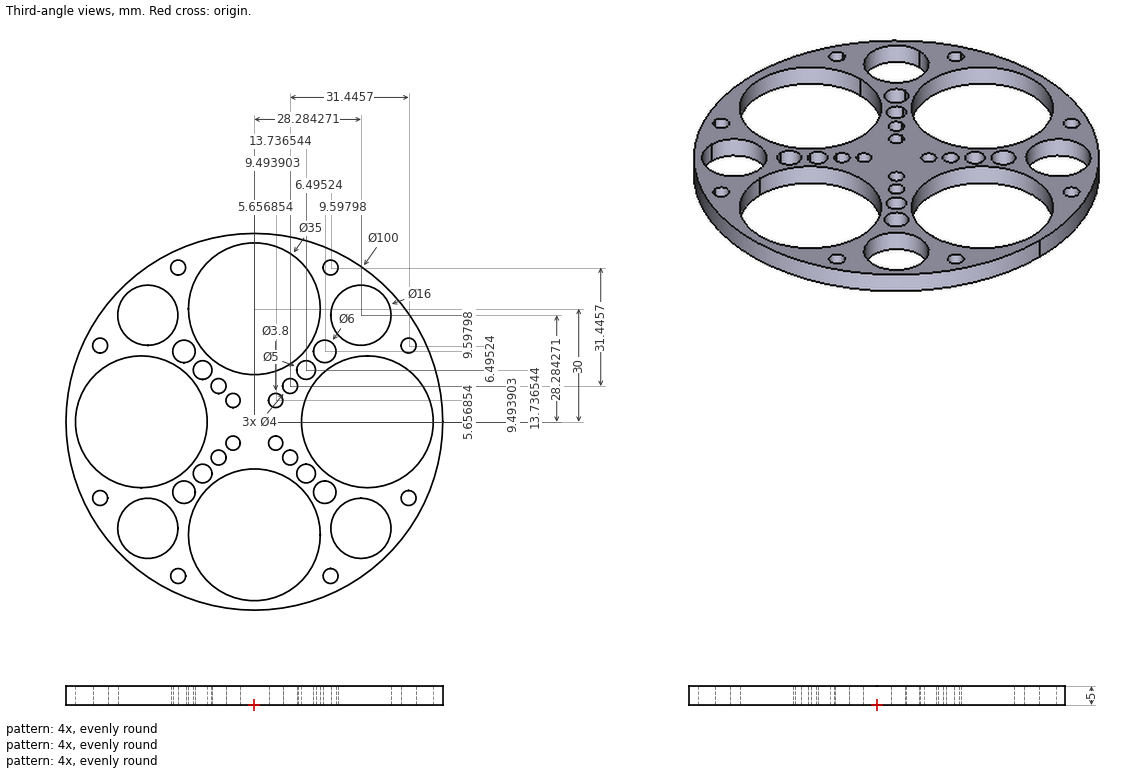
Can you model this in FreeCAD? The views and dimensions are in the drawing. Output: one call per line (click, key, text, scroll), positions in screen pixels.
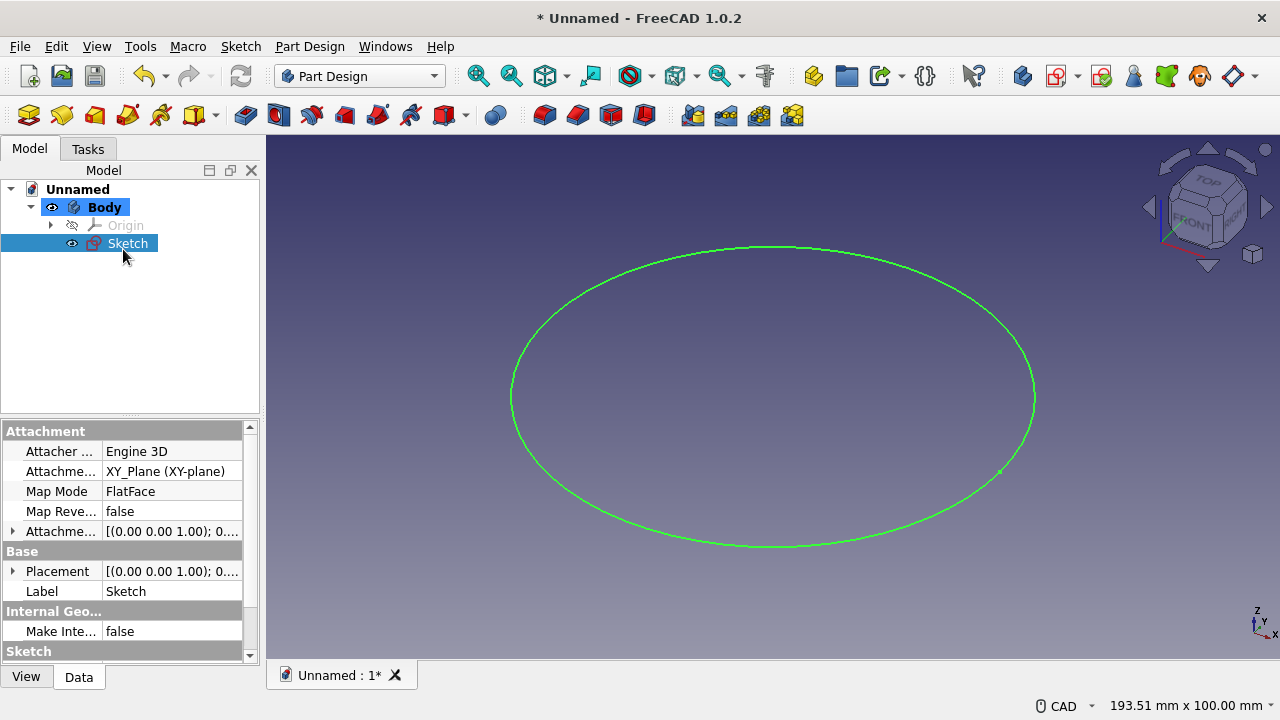
click(29, 116)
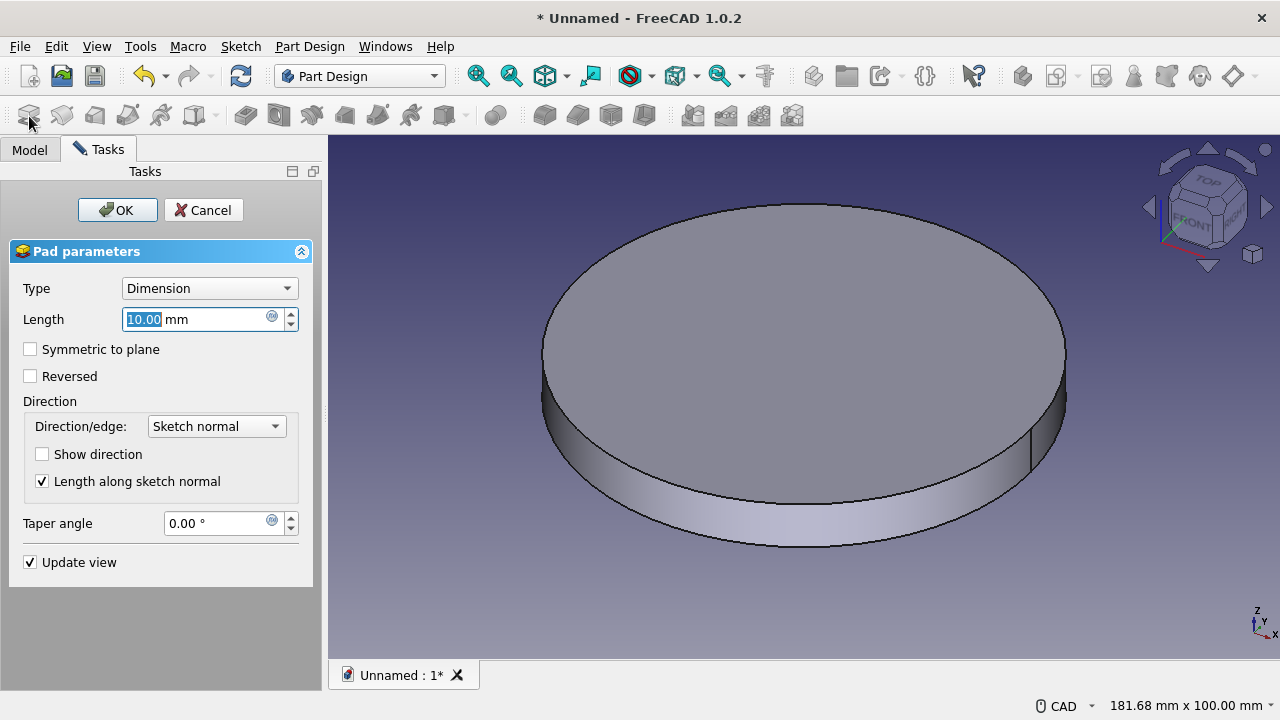
text(5)
key(Tab)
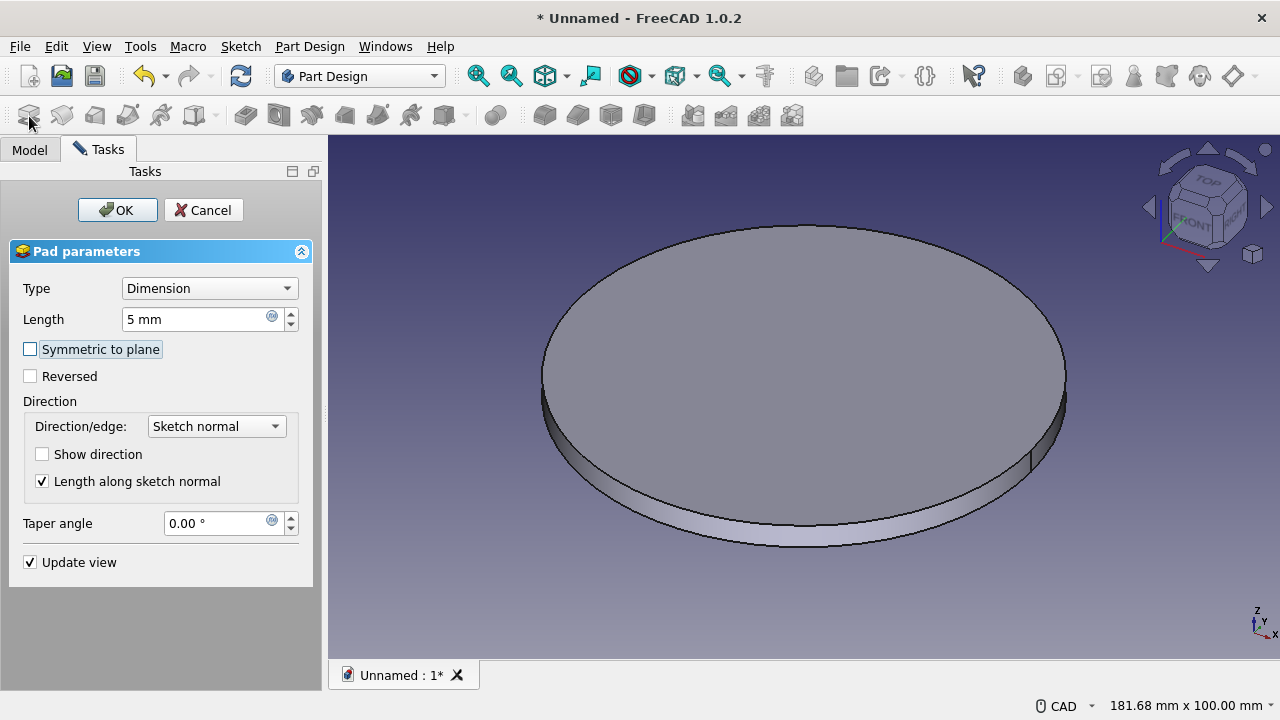
click(118, 210)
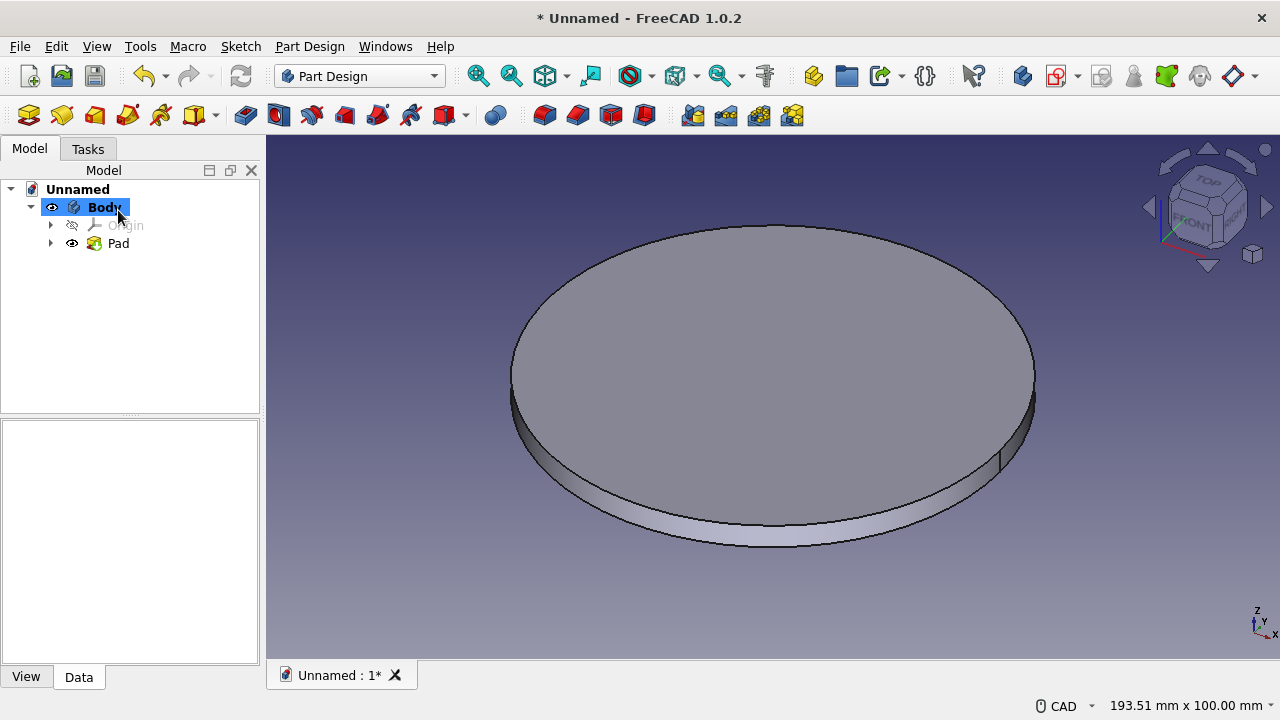
key(5)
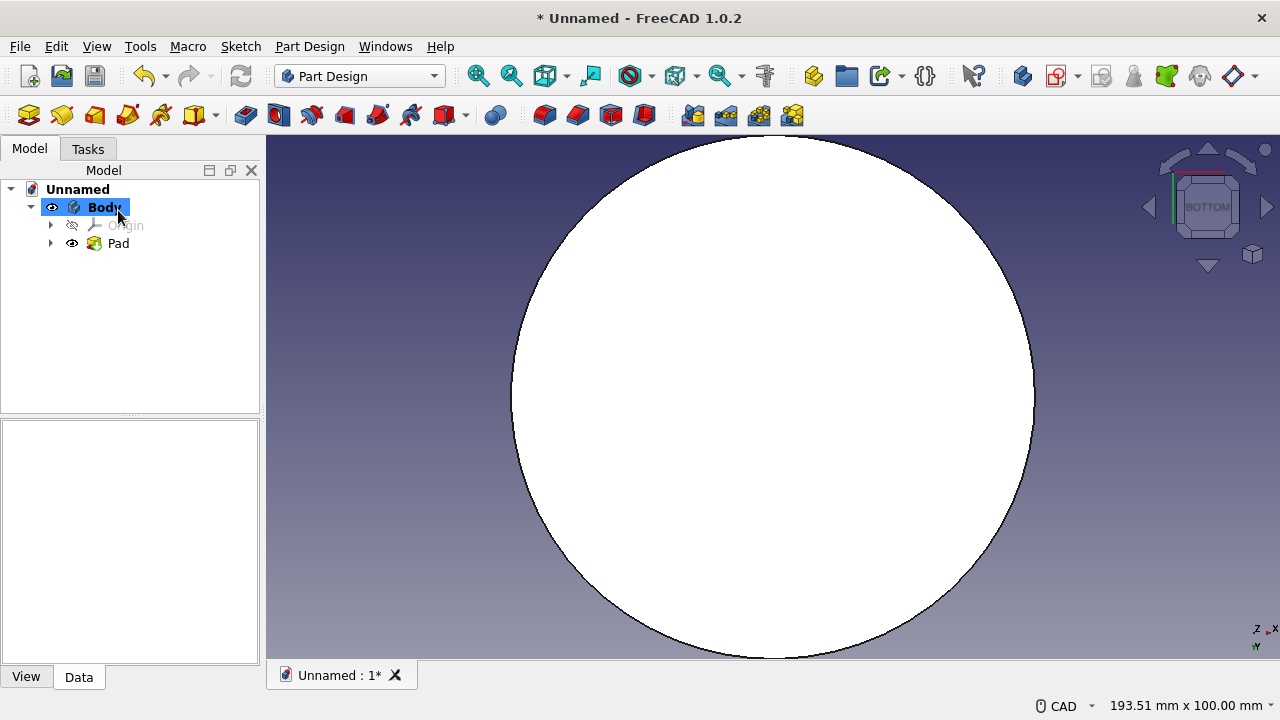
key(v)
key(f)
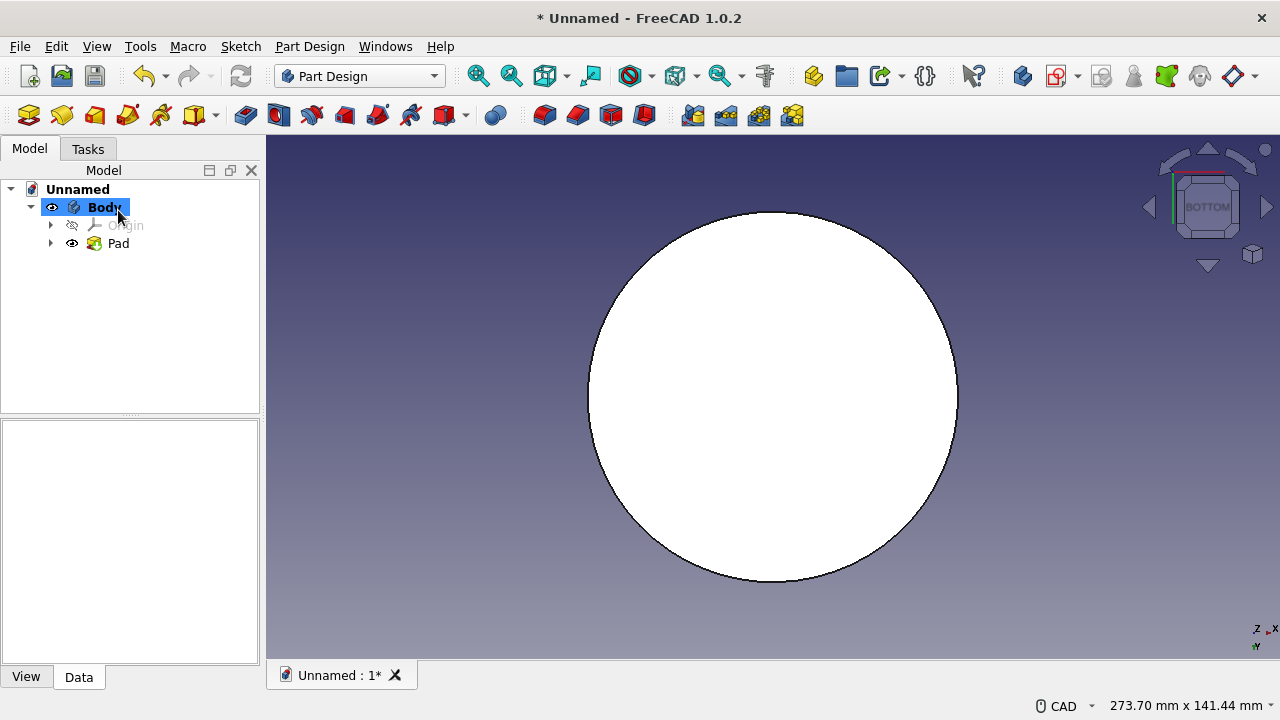
click(773, 396)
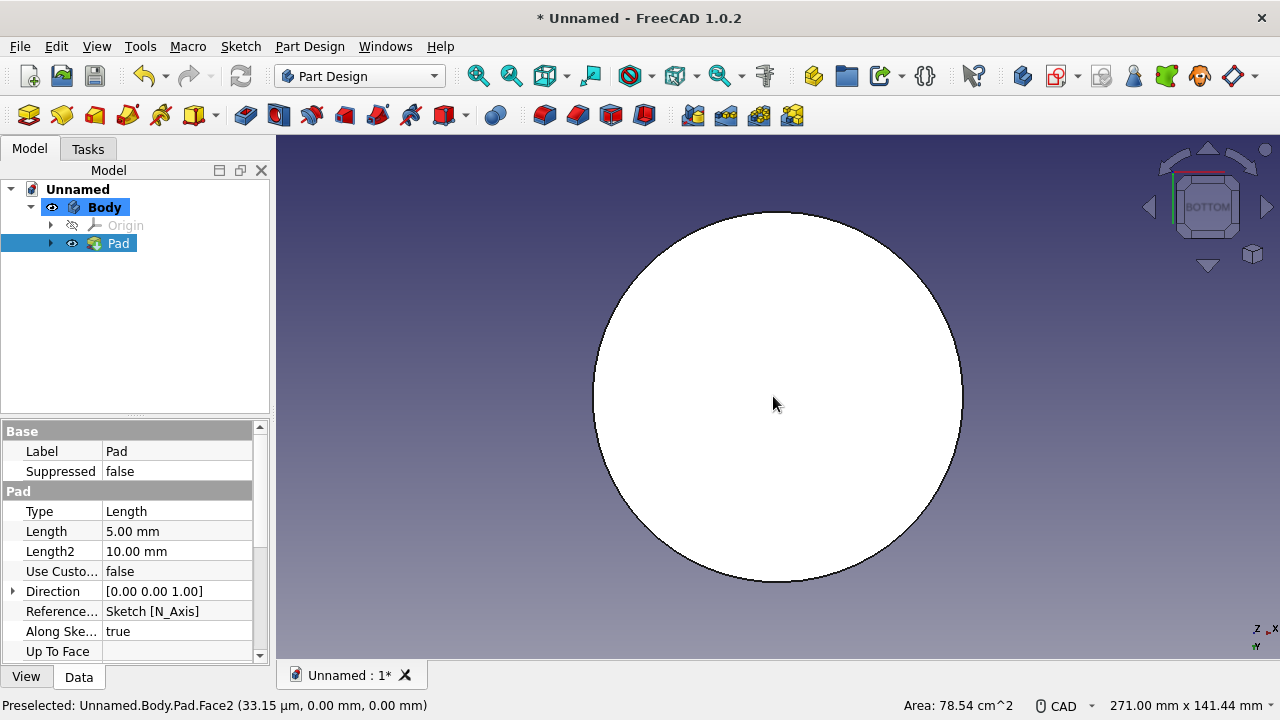
click(1056, 76)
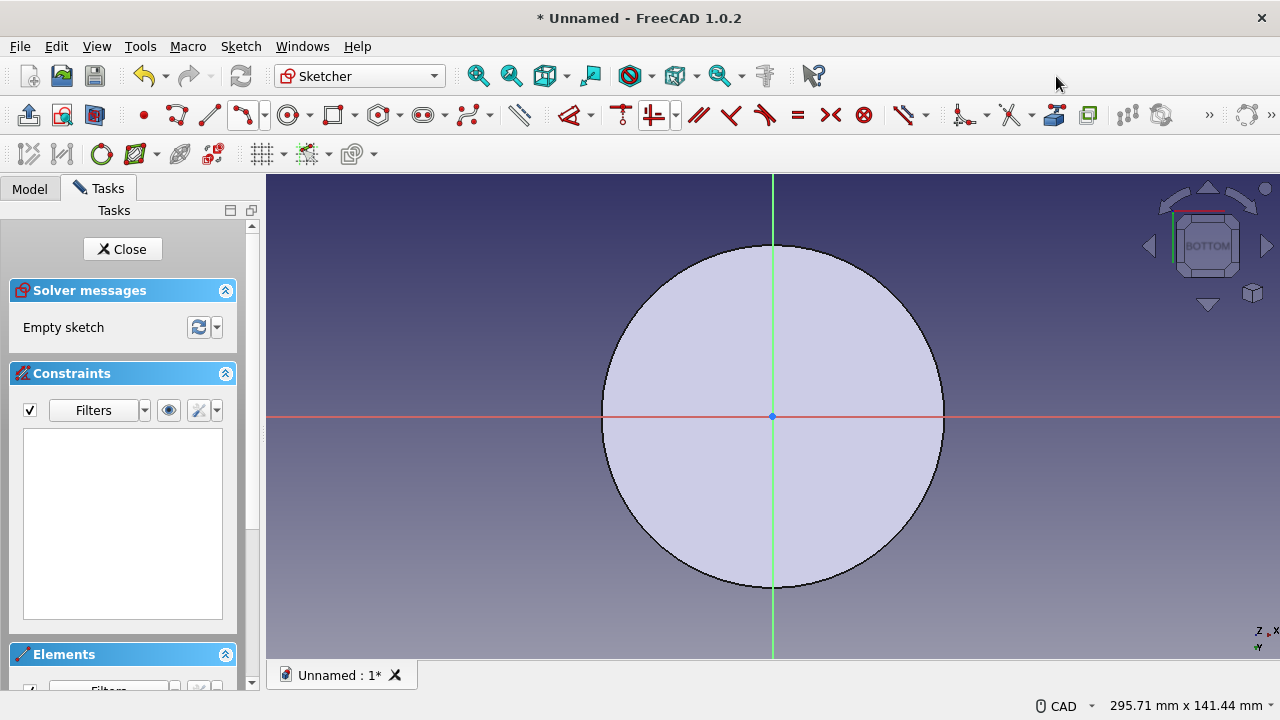
scroll(794, 431, up, 12)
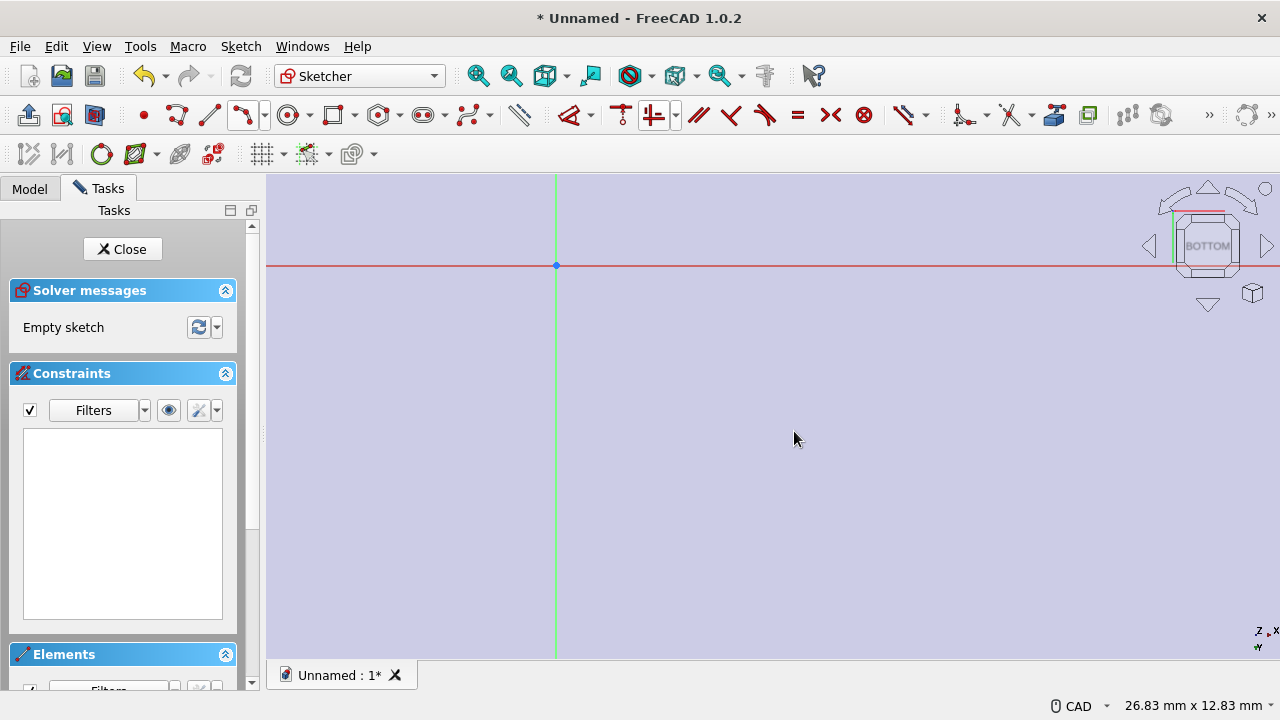
key(g)
key(c)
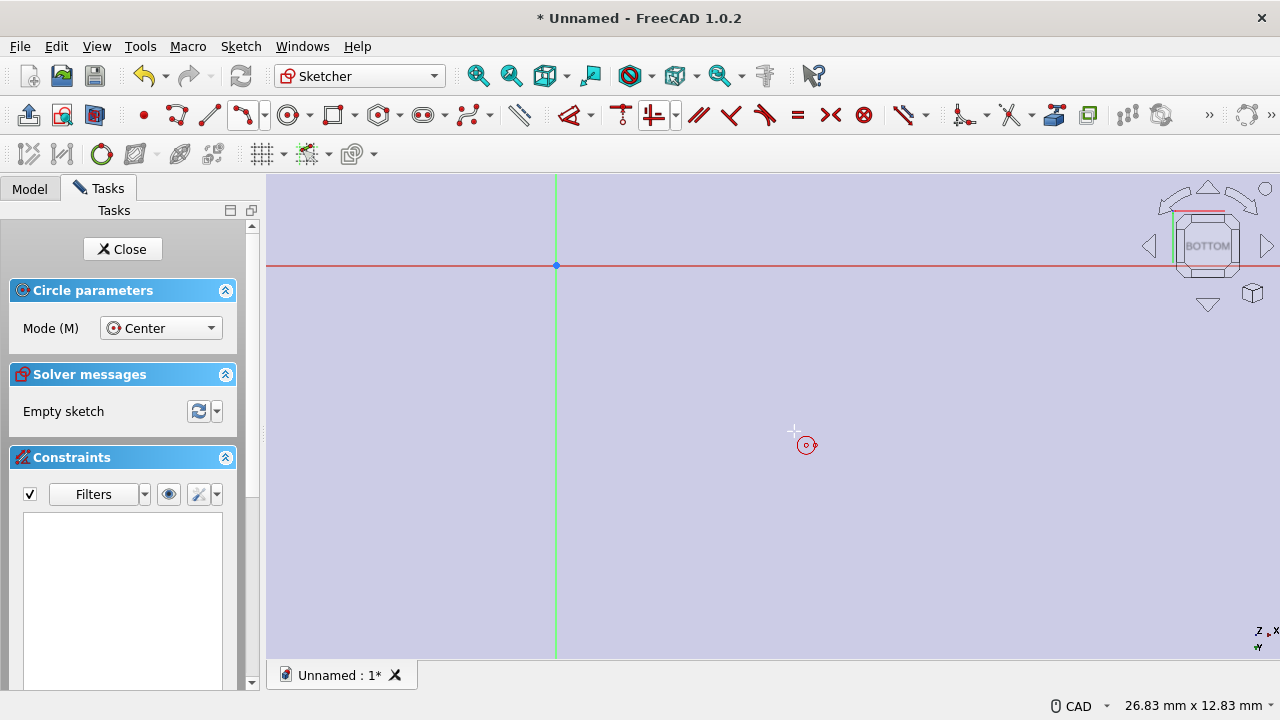
click(770, 480)
click(821, 429)
key(Escape)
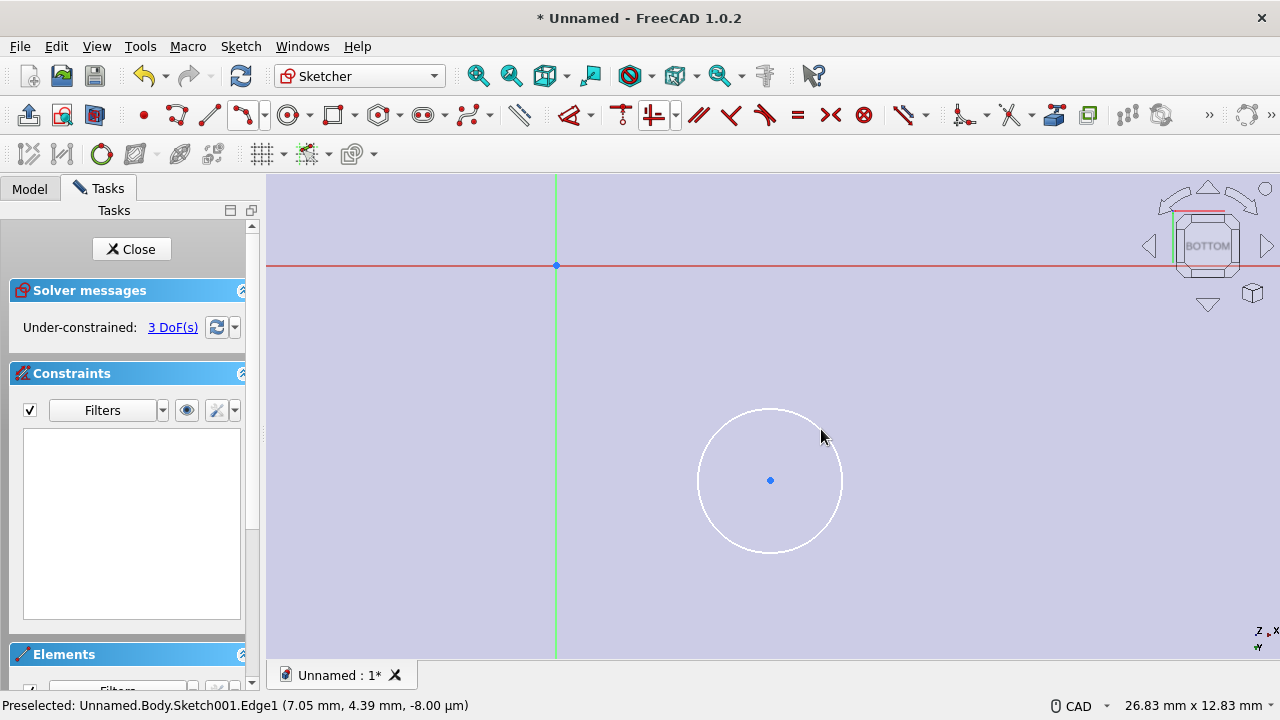
click(568, 116)